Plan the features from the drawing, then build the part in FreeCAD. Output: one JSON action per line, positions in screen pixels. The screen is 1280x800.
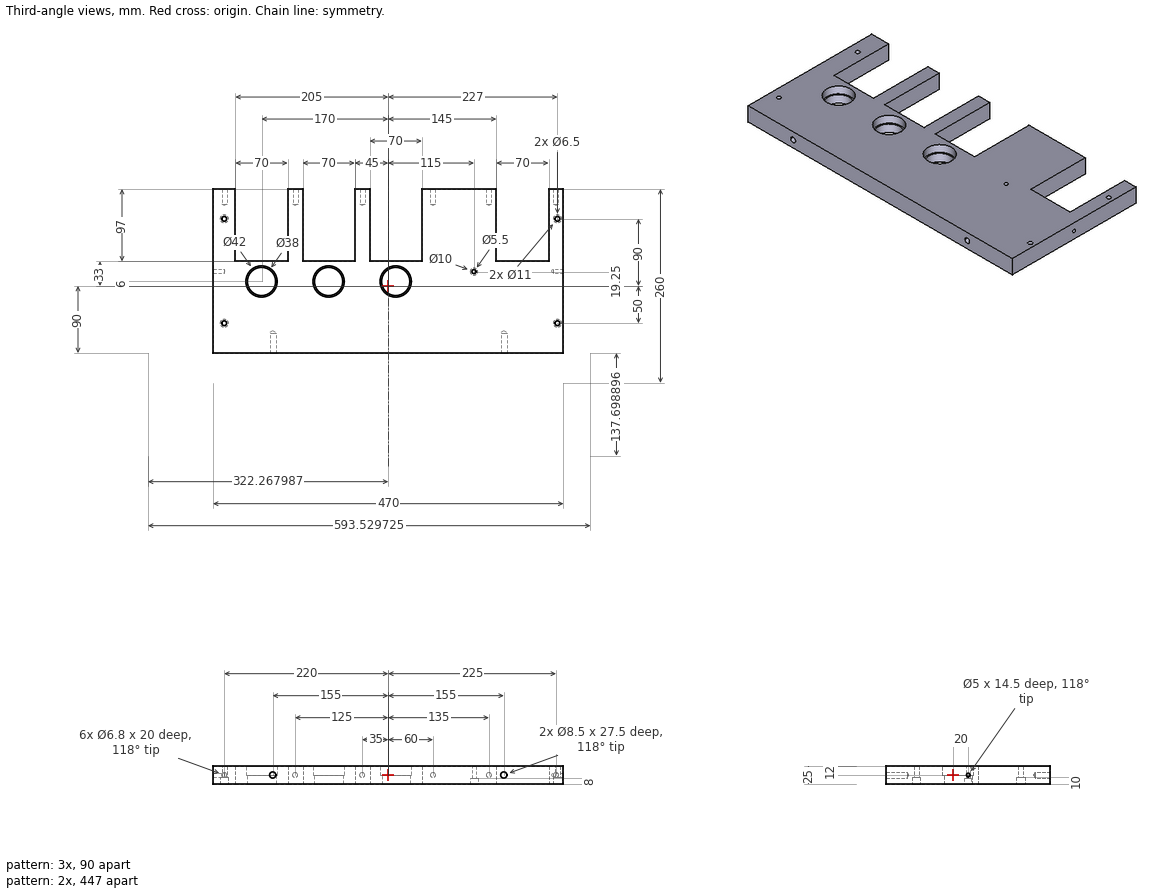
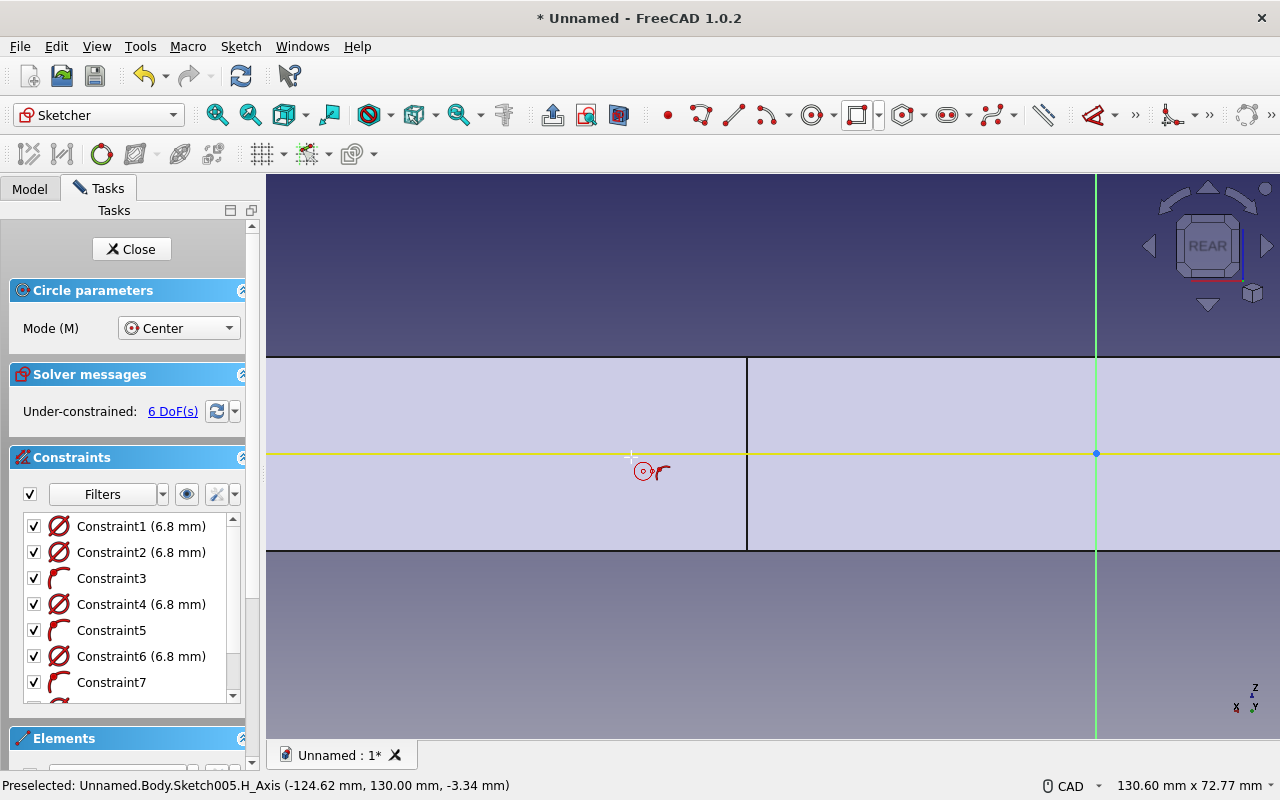
{"action": "scroll", "coordinate": [631, 457], "scroll_direction": "down", "scroll_amount": 9}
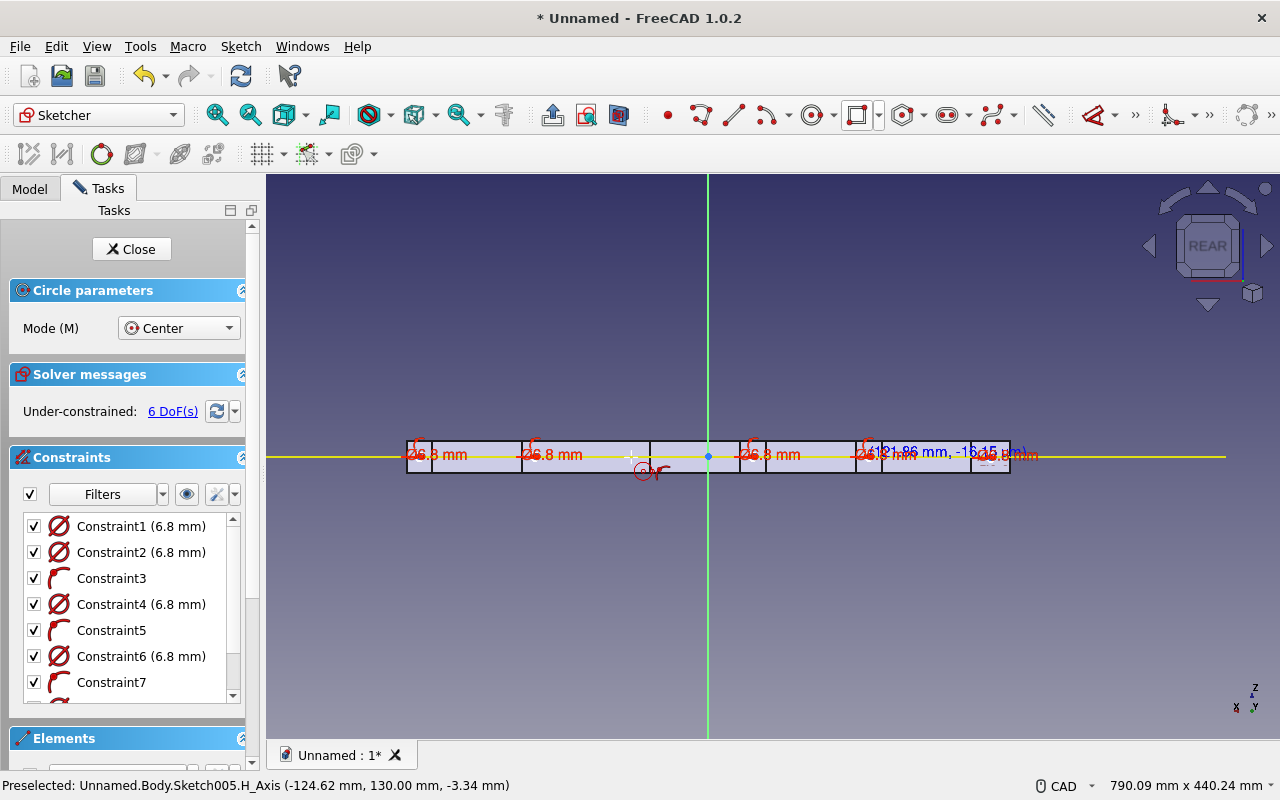
{"action": "left_click", "coordinate": [631, 457]}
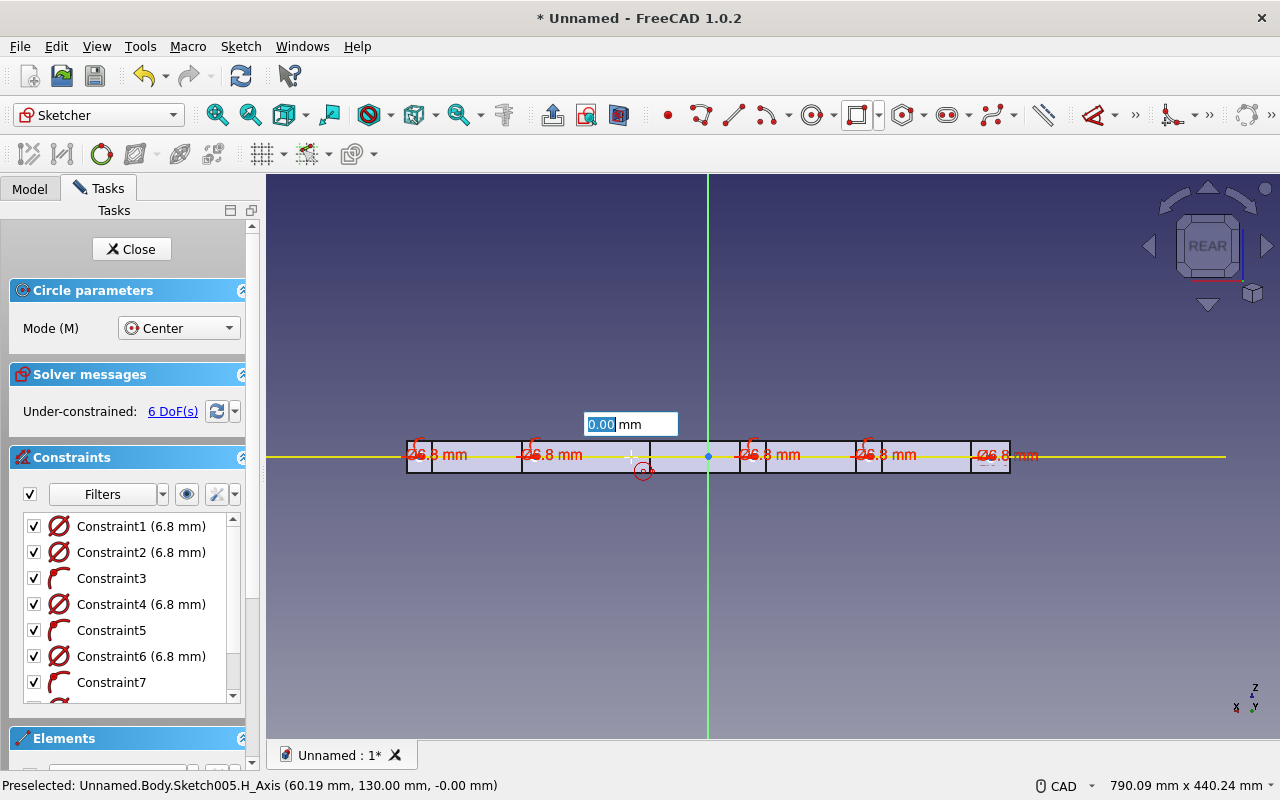
{"action": "scroll", "coordinate": [633, 453], "scroll_direction": "up", "scroll_amount": 7}
{"action": "mouse_move", "coordinate": [631, 451]}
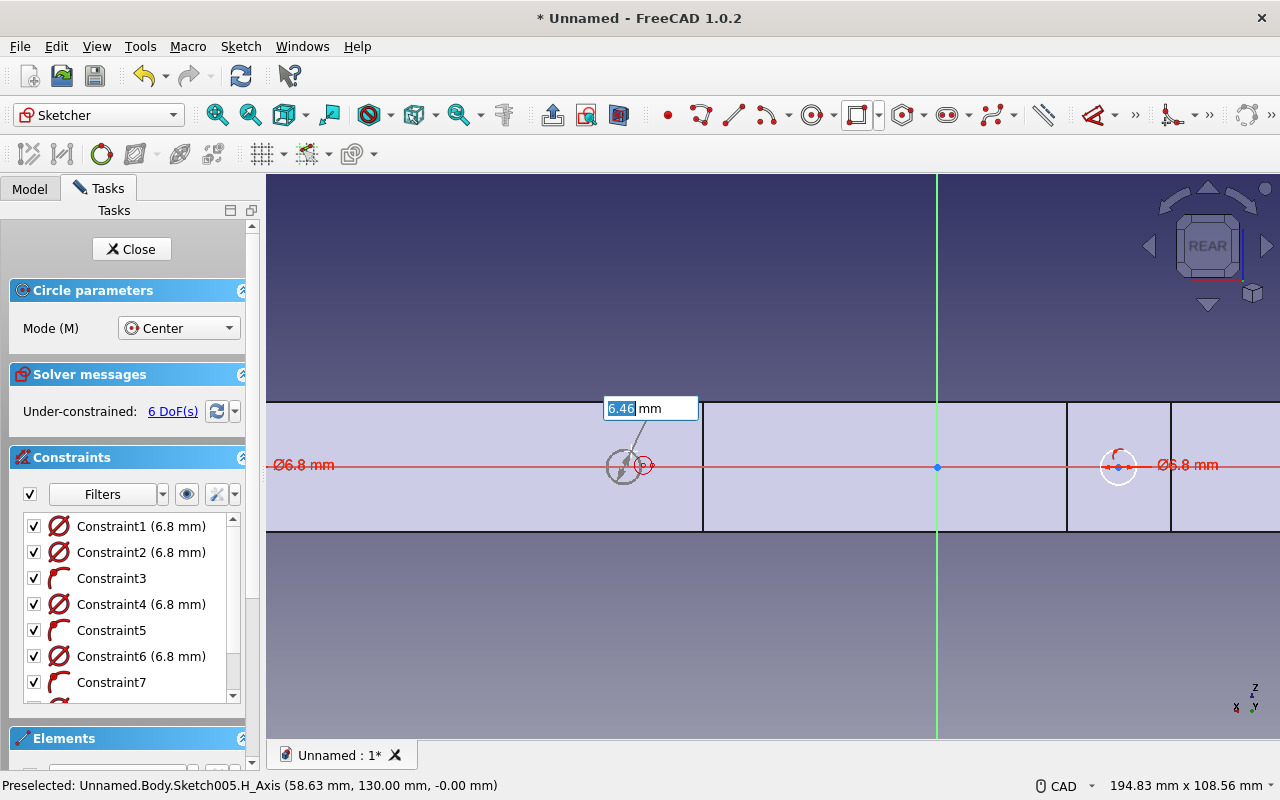
{"action": "type", "text": "6.8"}
{"action": "key", "text": "Return"}
{"action": "key", "text": "Escape"}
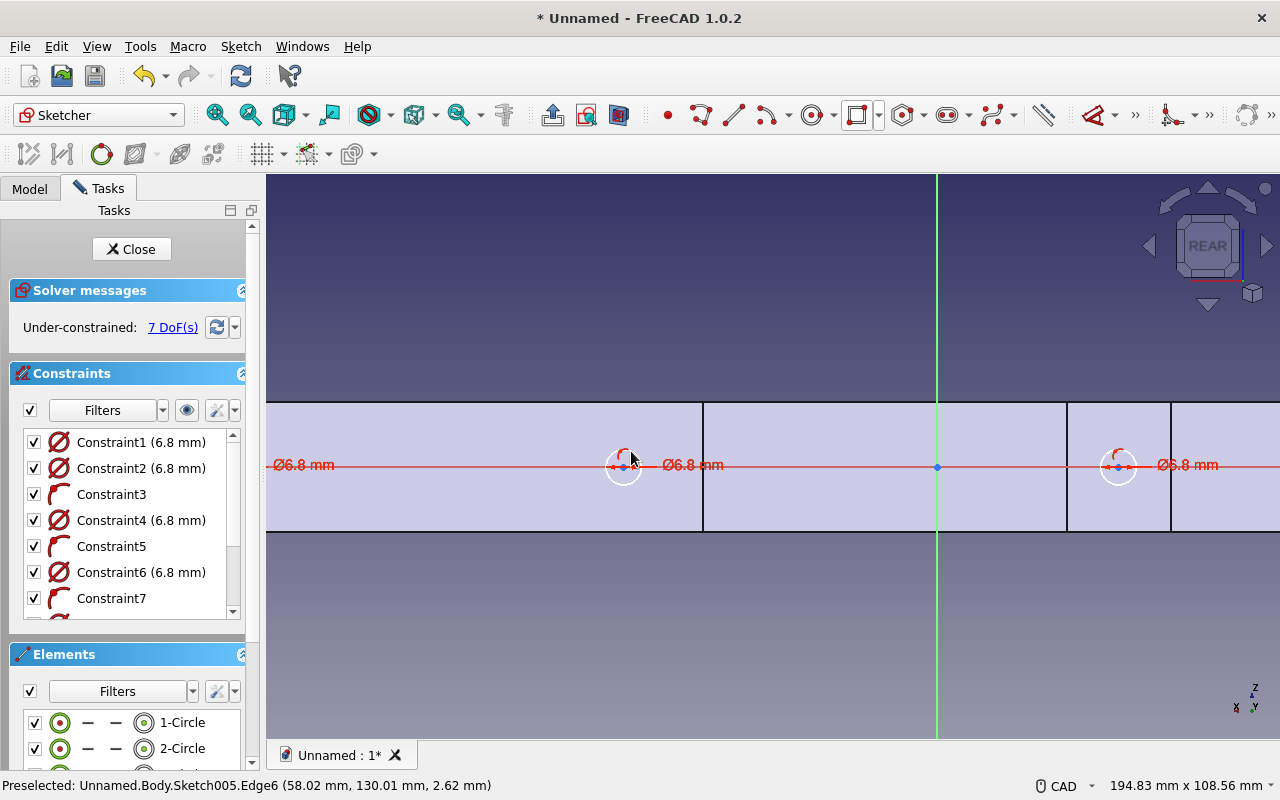
{"action": "scroll", "coordinate": [633, 453], "scroll_direction": "down", "scroll_amount": 7}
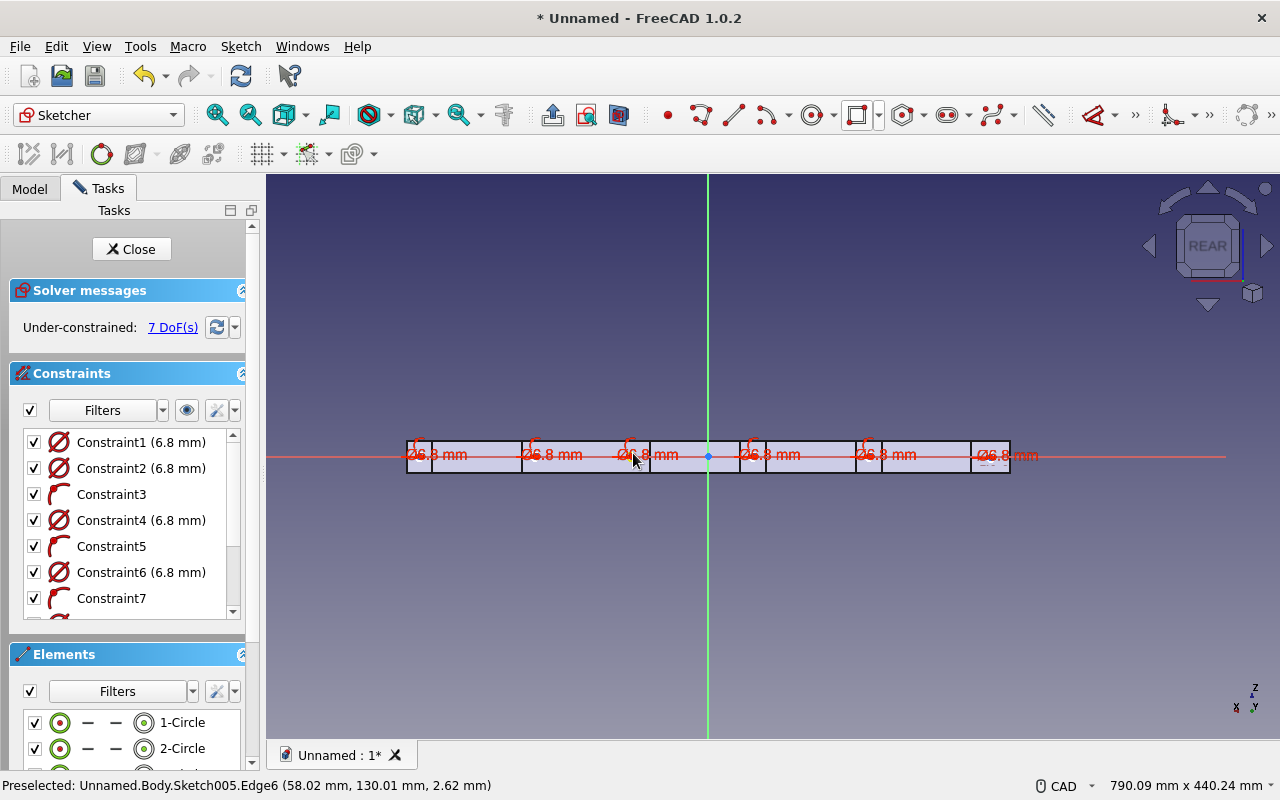
{"action": "left_click", "coordinate": [991, 458]}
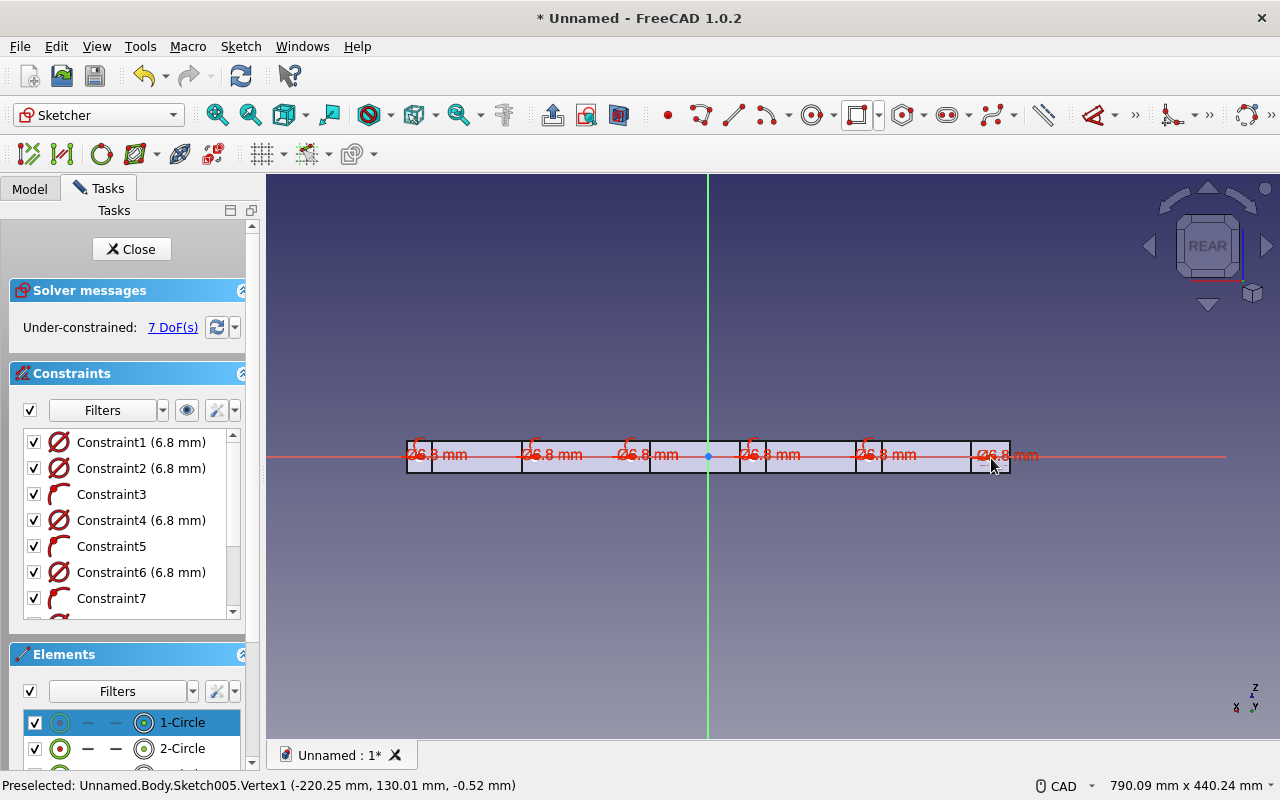
{"action": "left_click", "coordinate": [353, 457]}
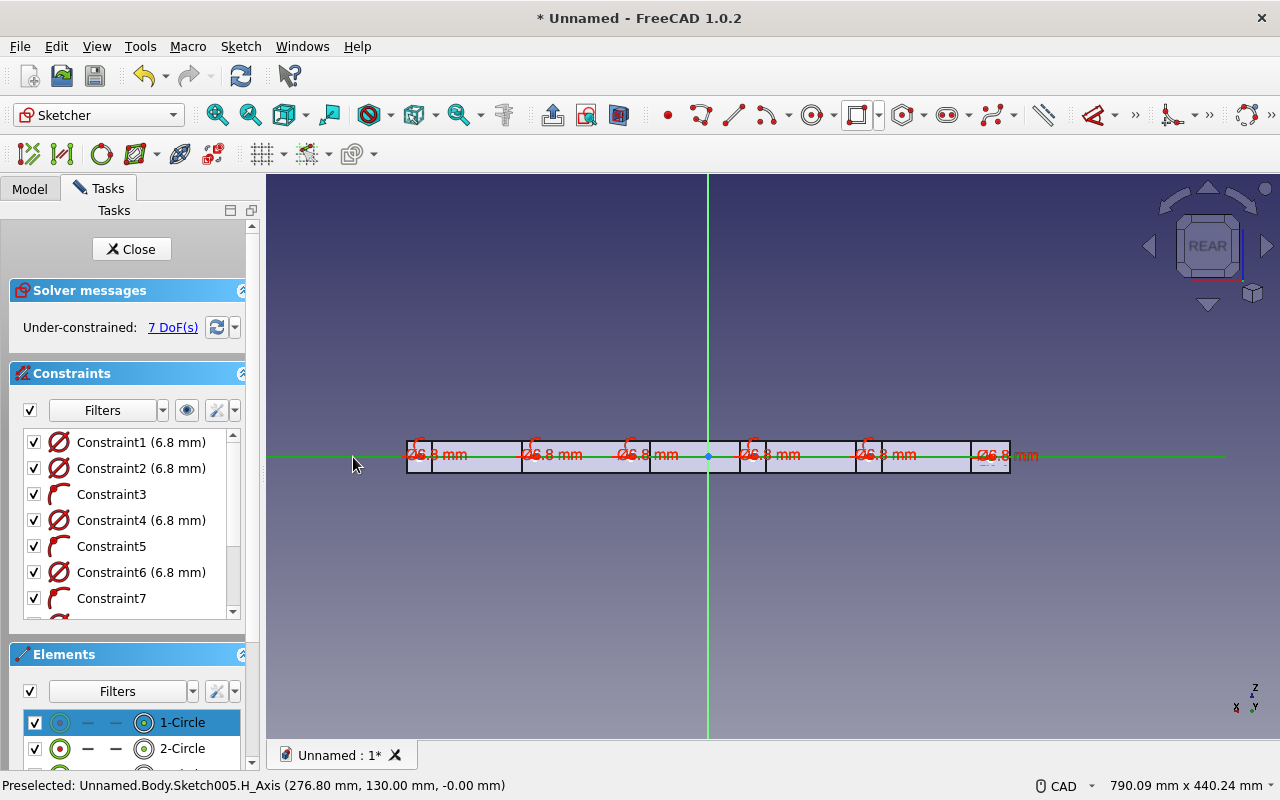
{"action": "key", "text": "c"}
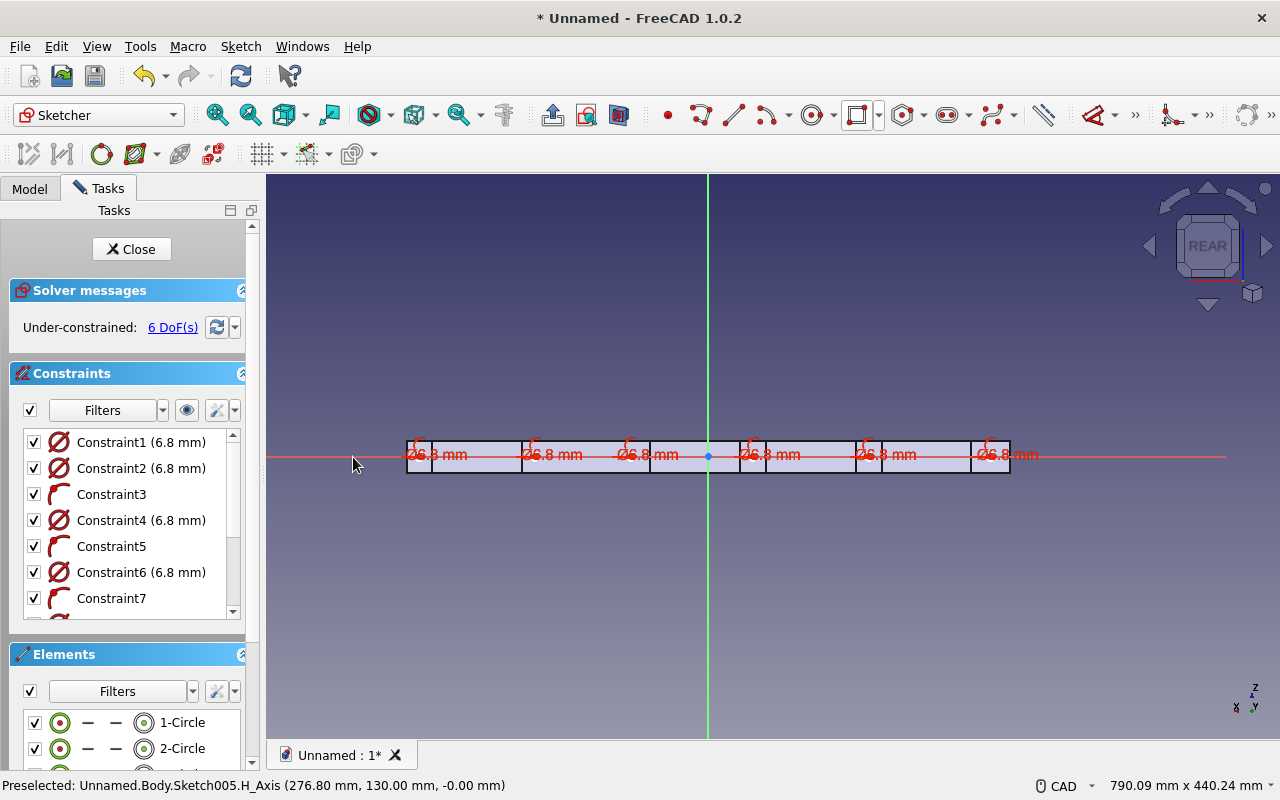
{"action": "left_click", "coordinate": [1092, 116]}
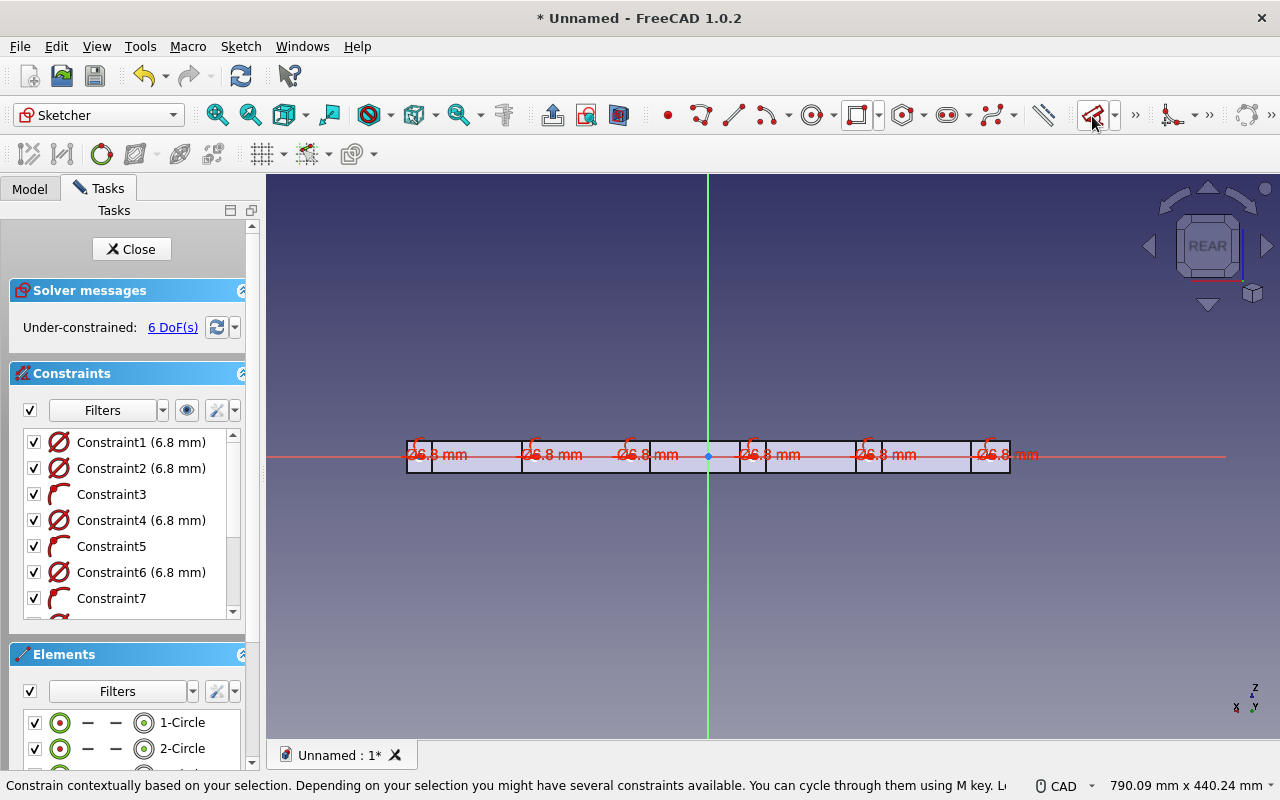
{"action": "left_click", "coordinate": [753, 457]}
{"action": "left_click", "coordinate": [731, 491]}